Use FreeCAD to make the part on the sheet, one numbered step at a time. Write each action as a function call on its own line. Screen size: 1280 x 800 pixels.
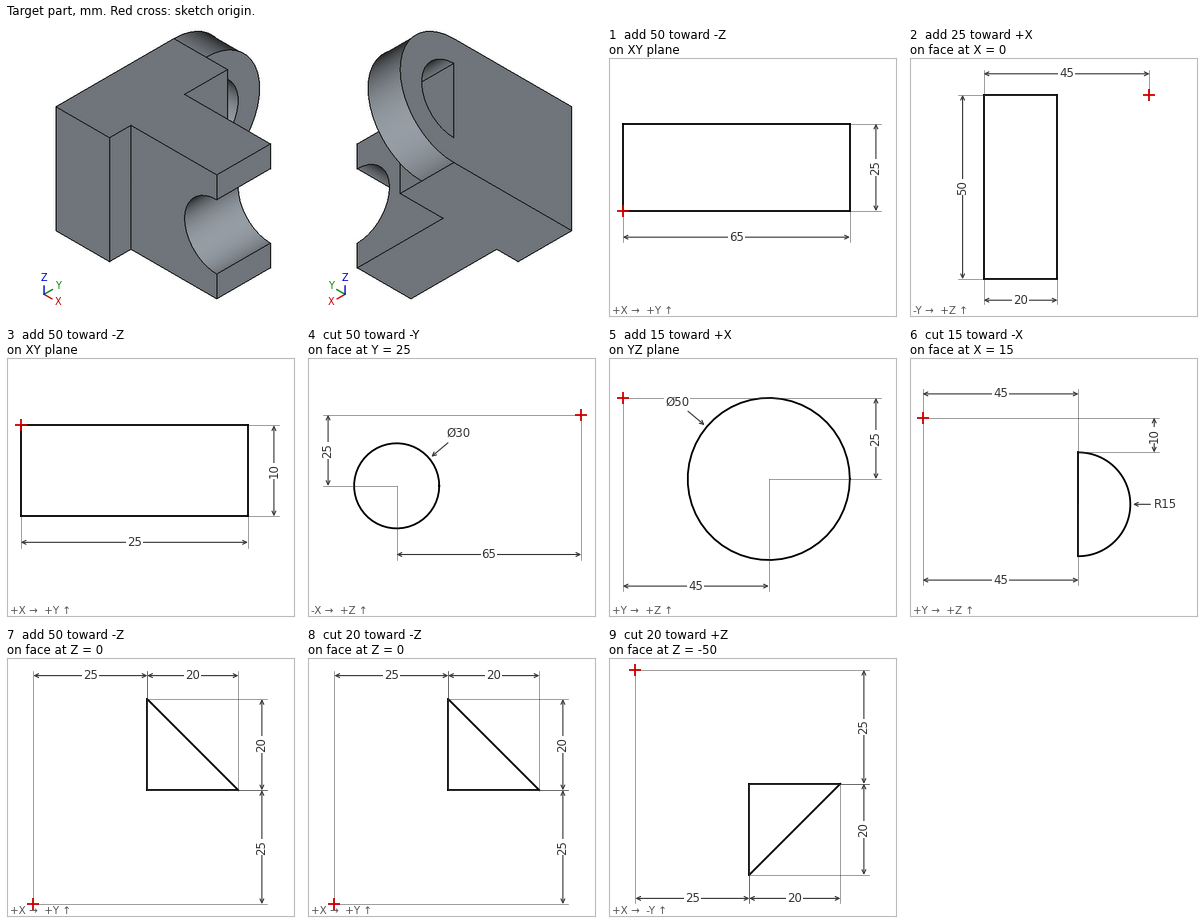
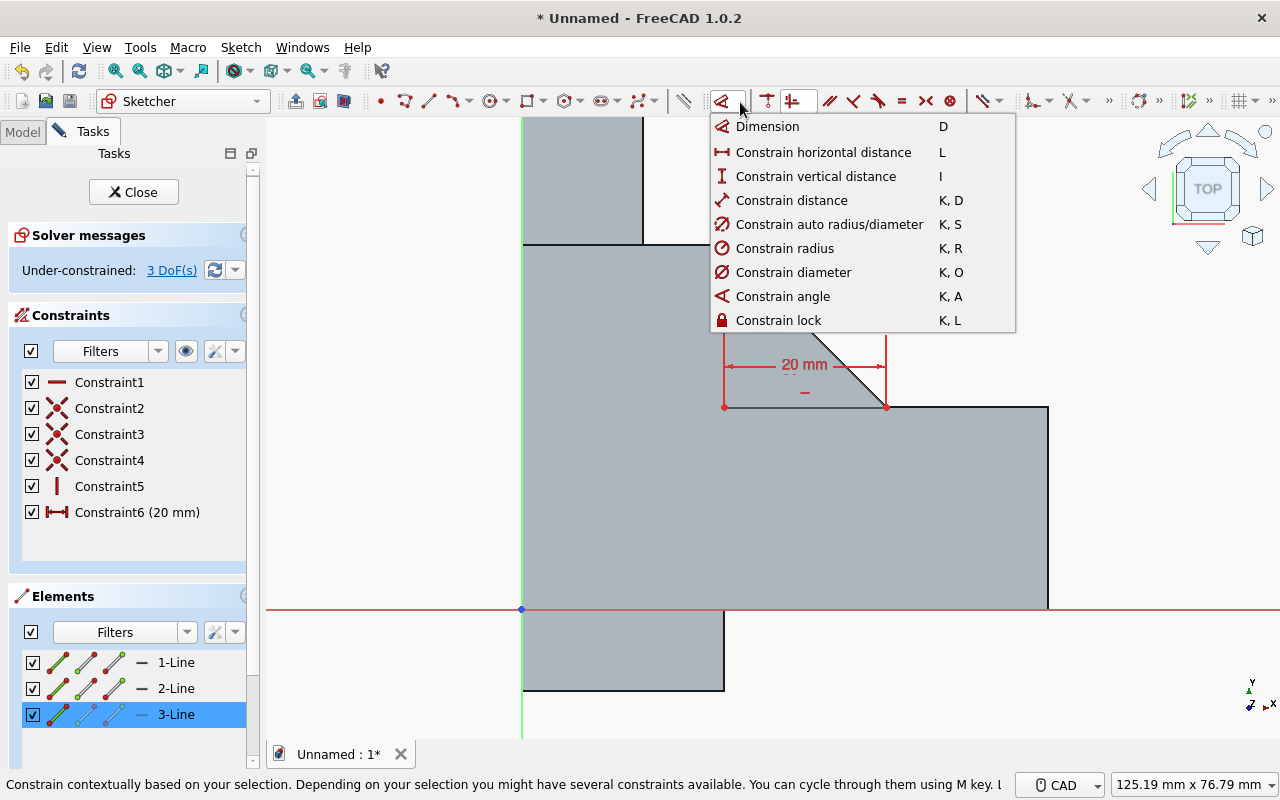
click(863, 176)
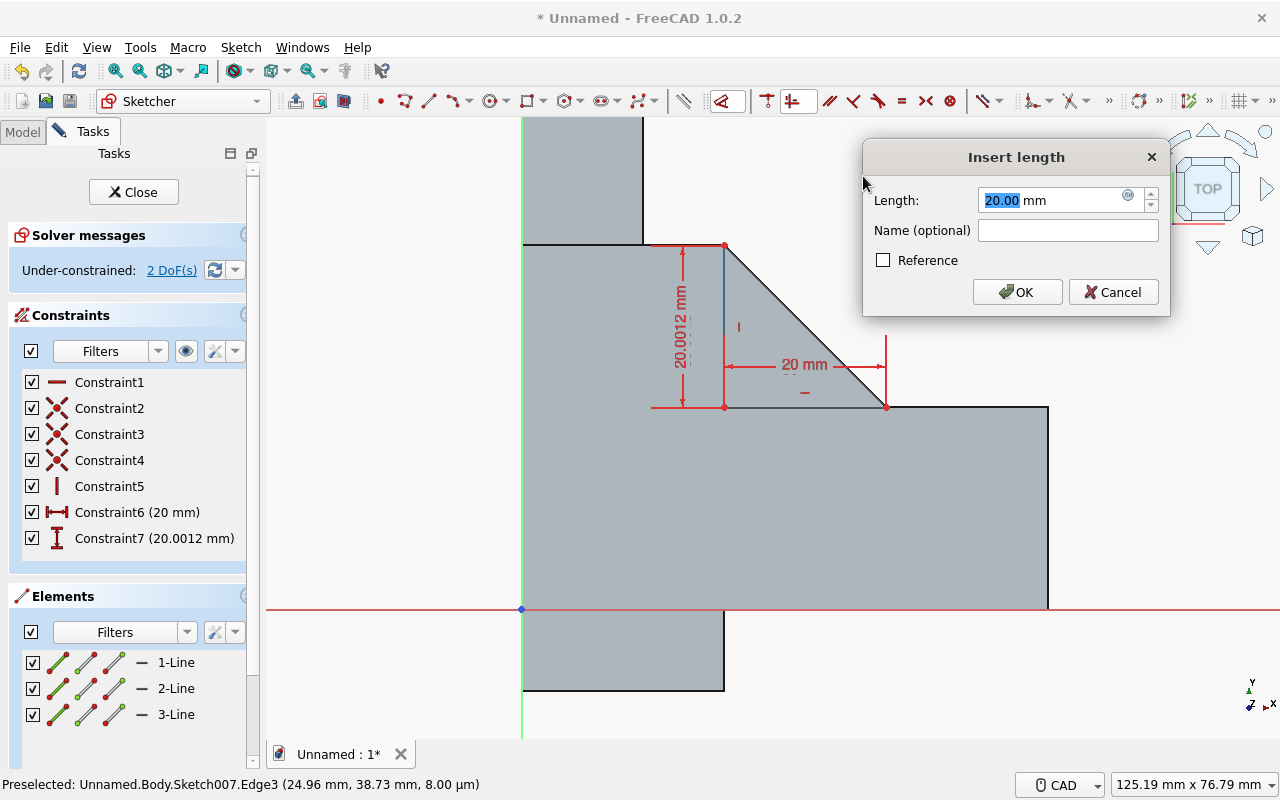
text(20)
key(Return)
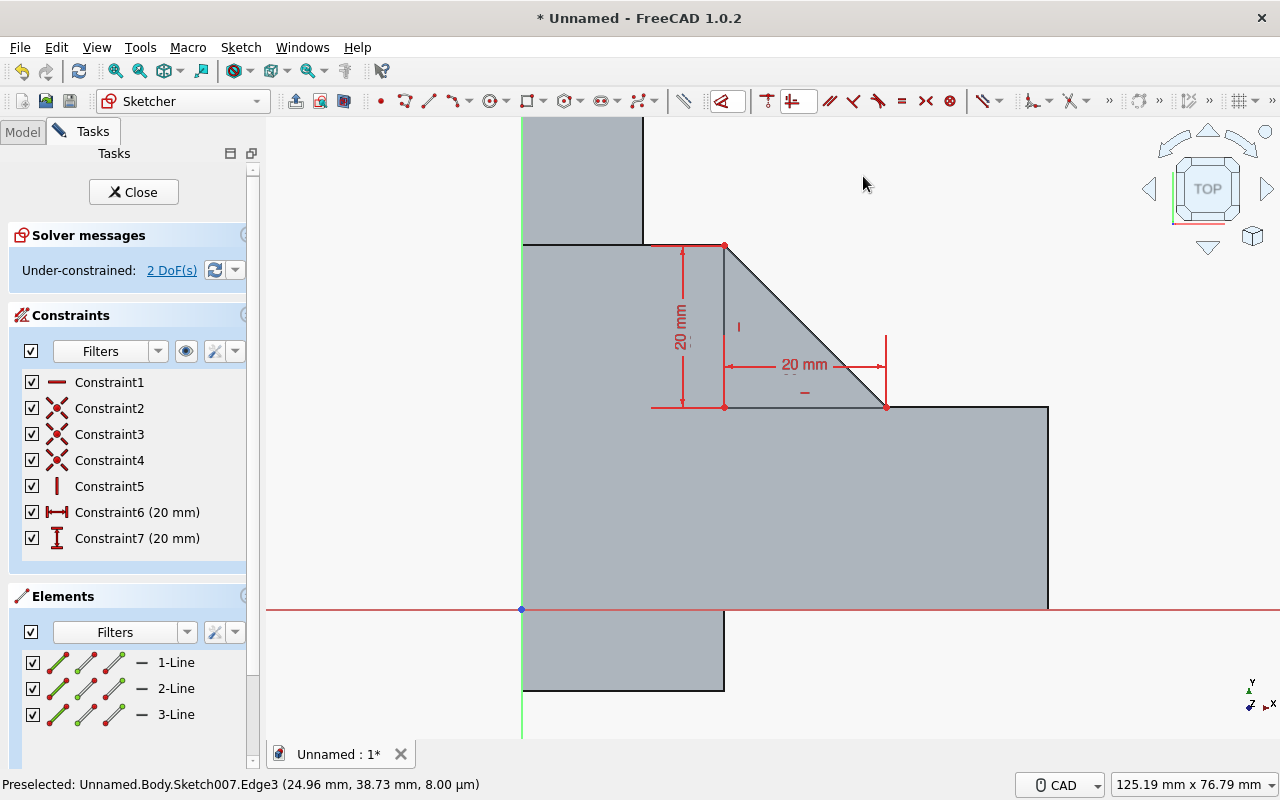
click(724, 408)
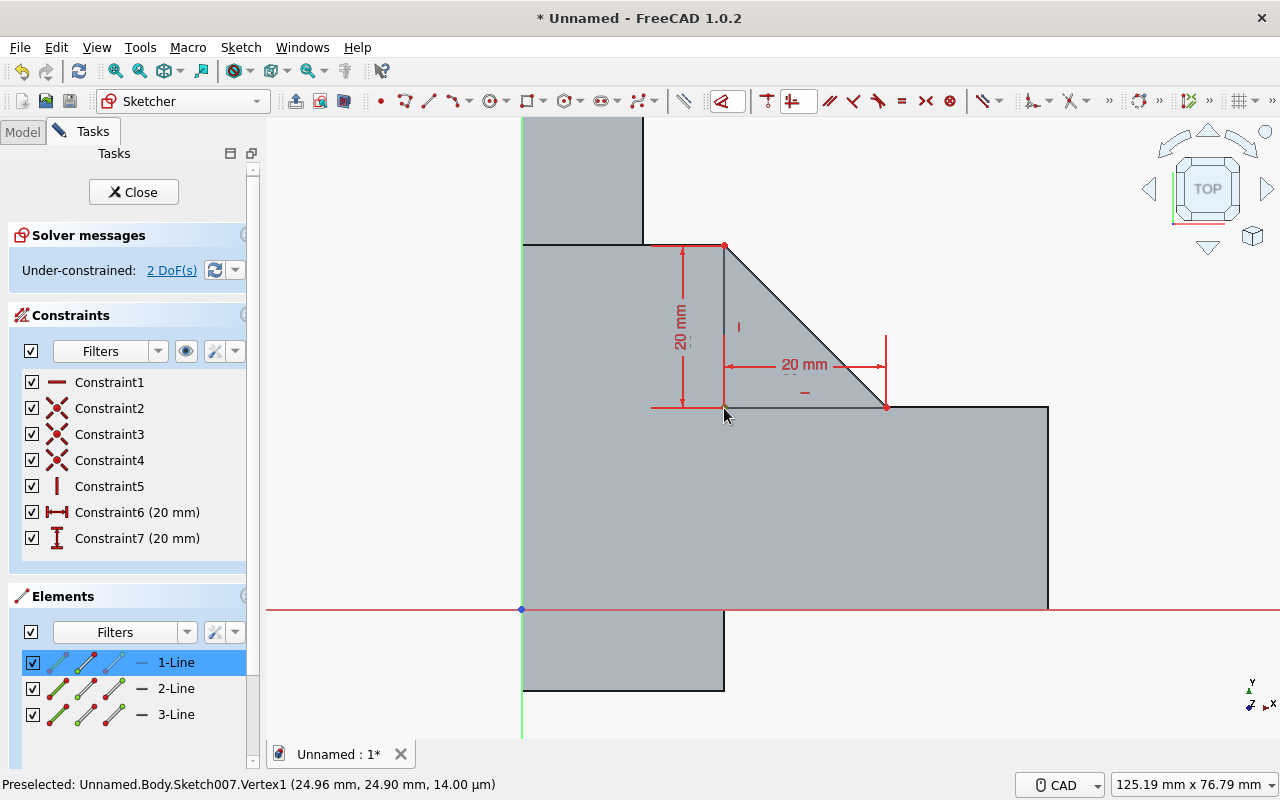
click(740, 102)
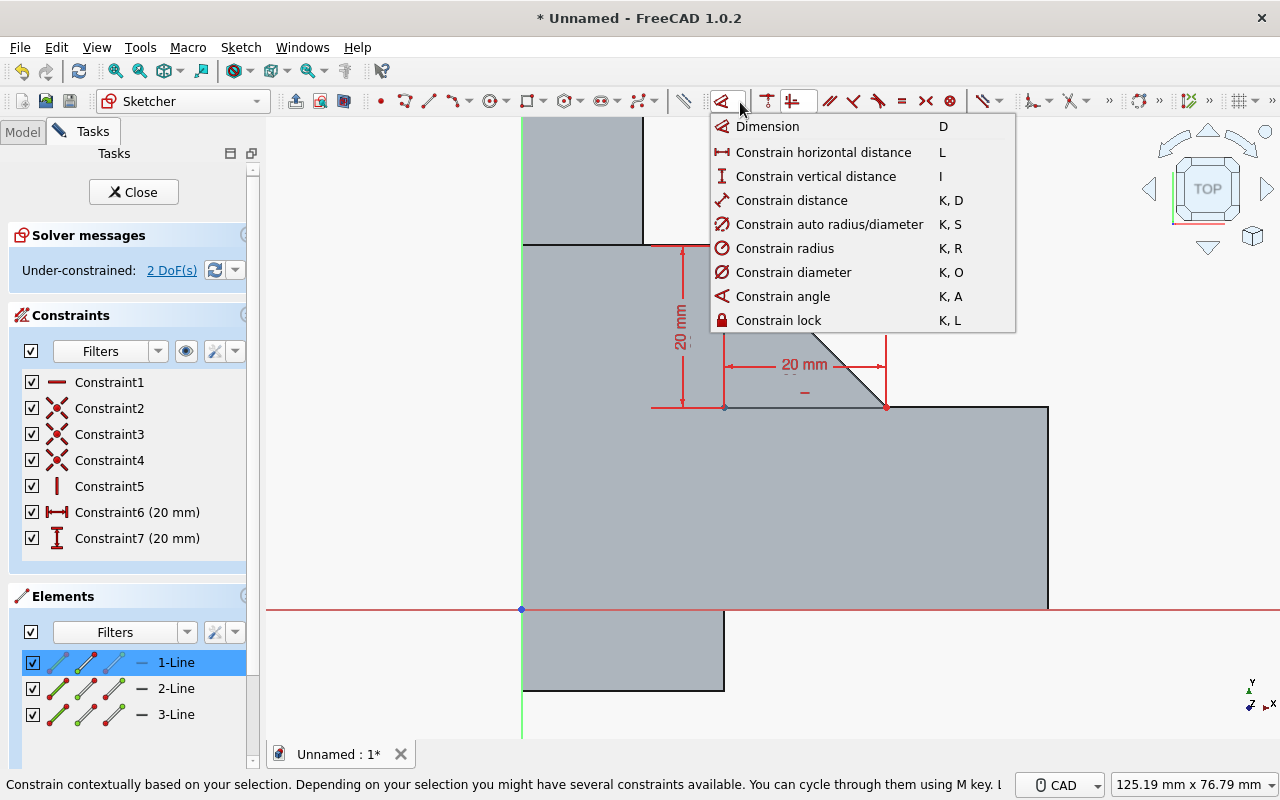
click(863, 152)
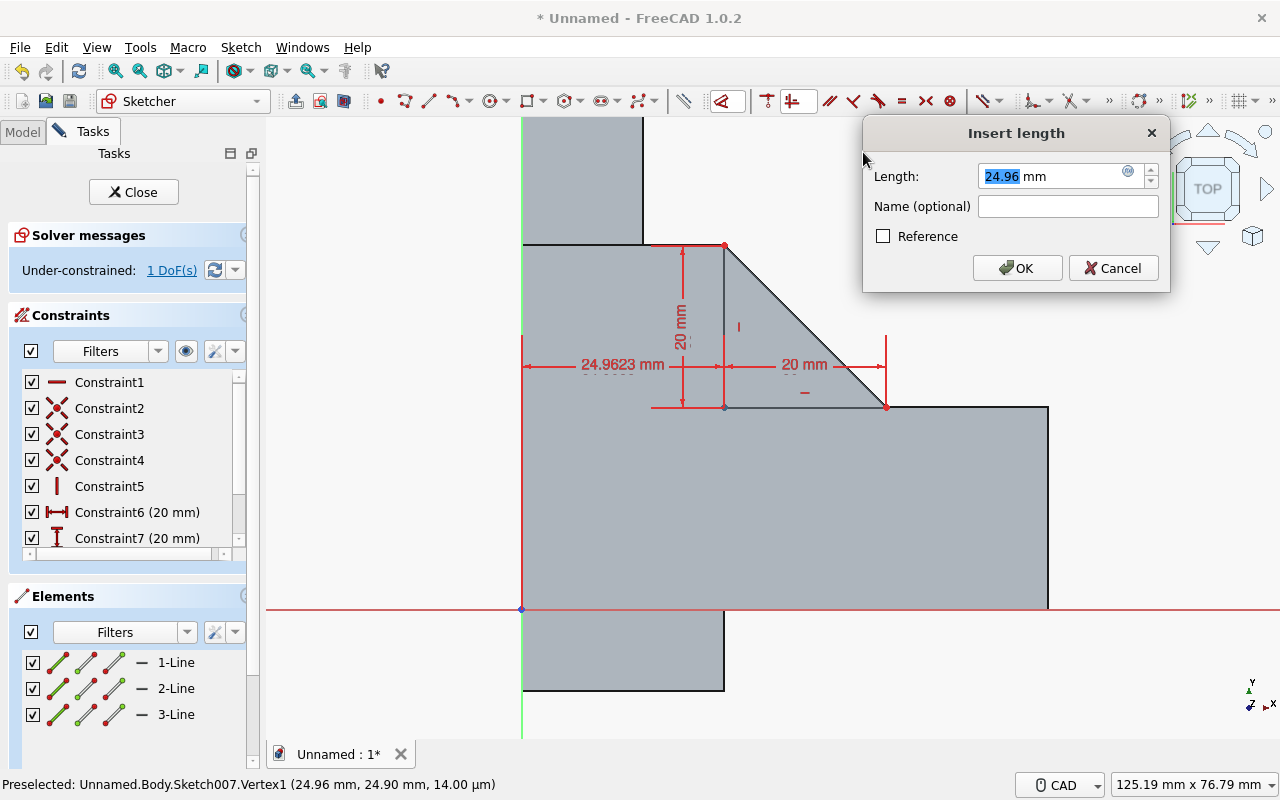
text(25)
key(Return)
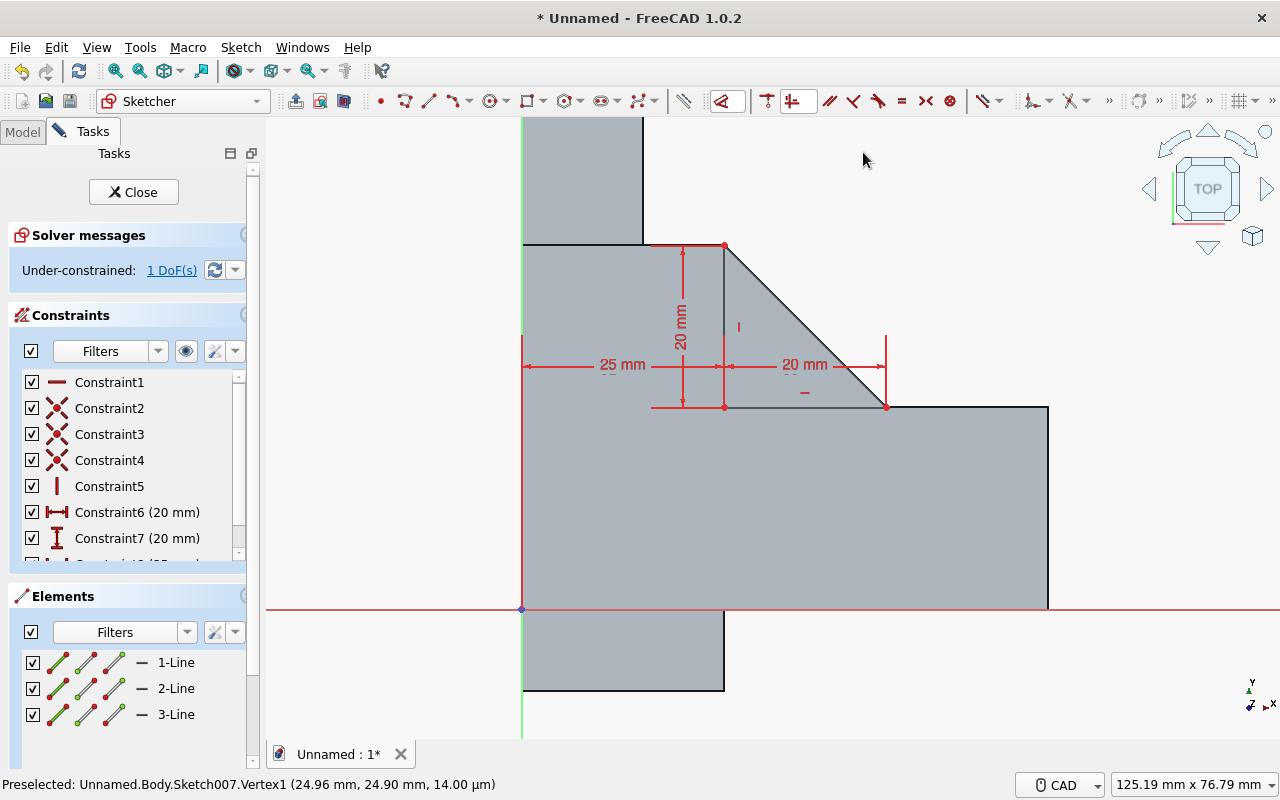
click(724, 408)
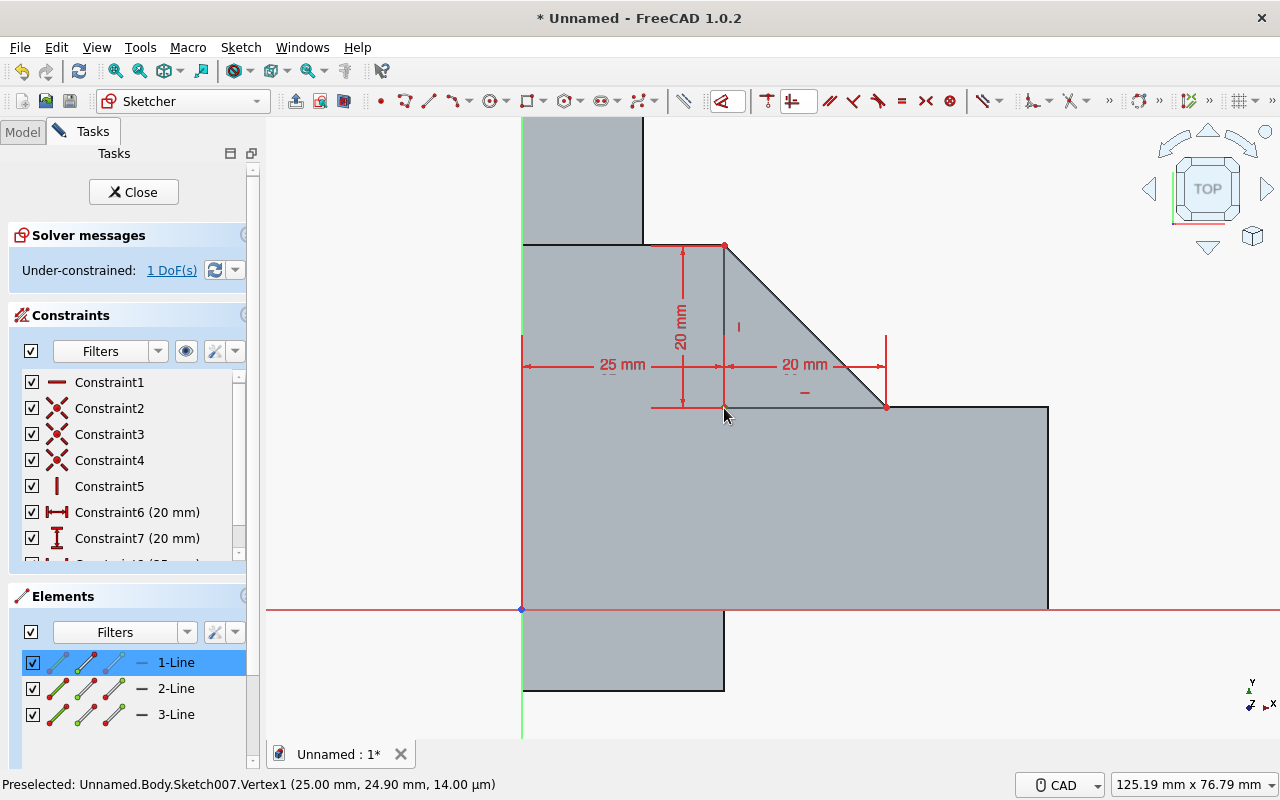
click(740, 102)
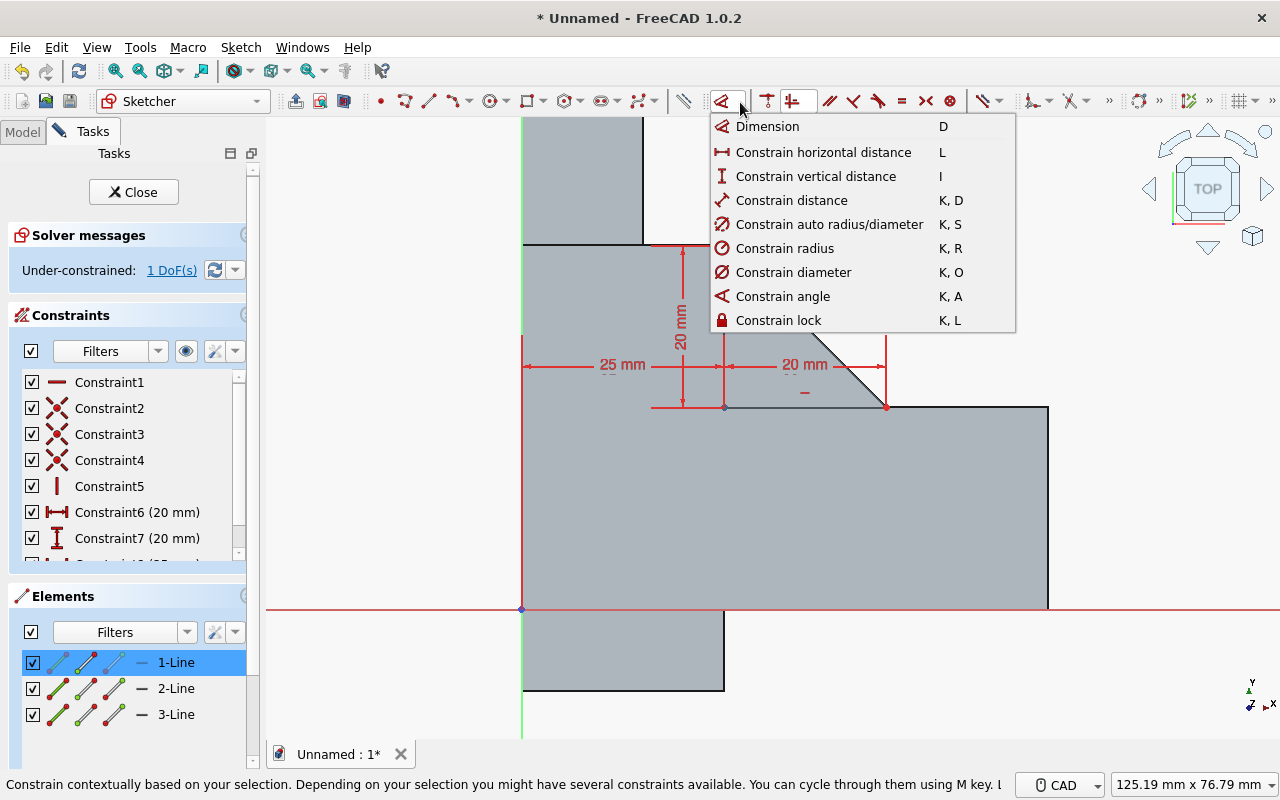
click(863, 176)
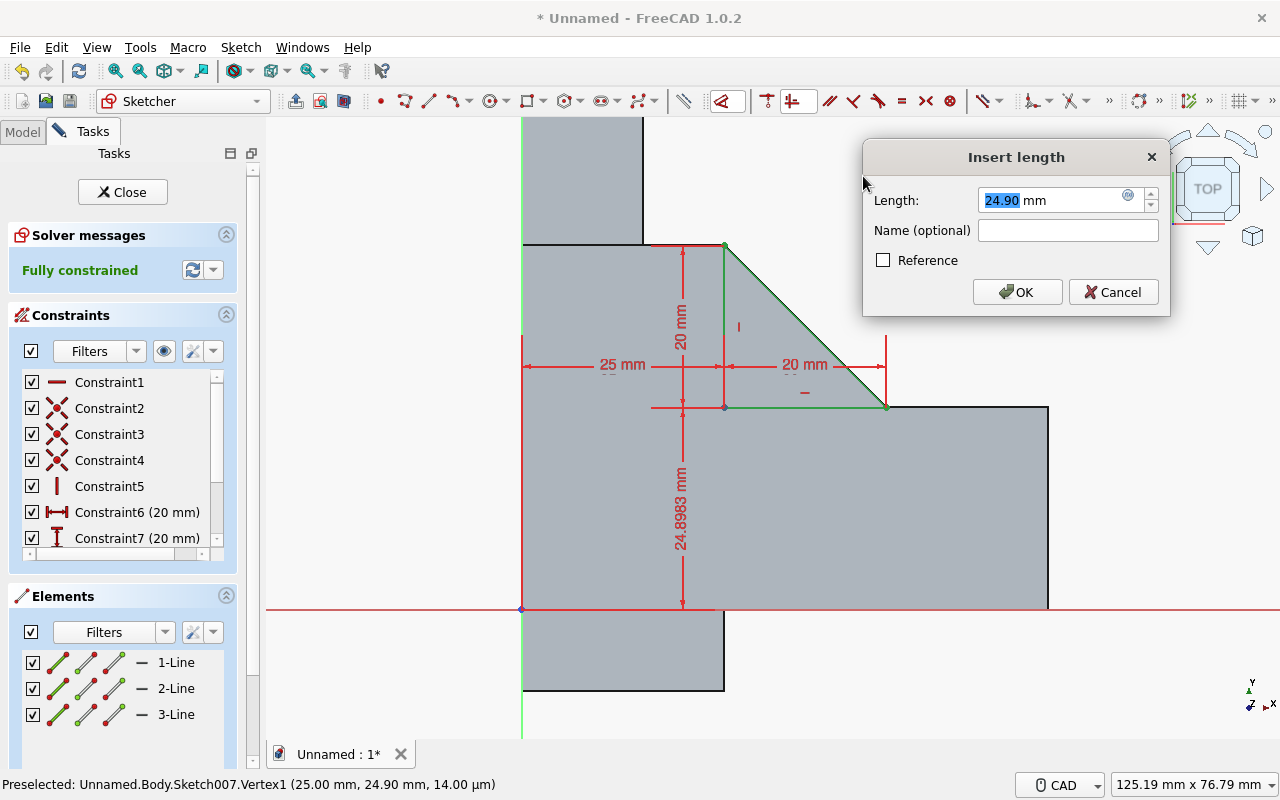
text(25)
key(Return)